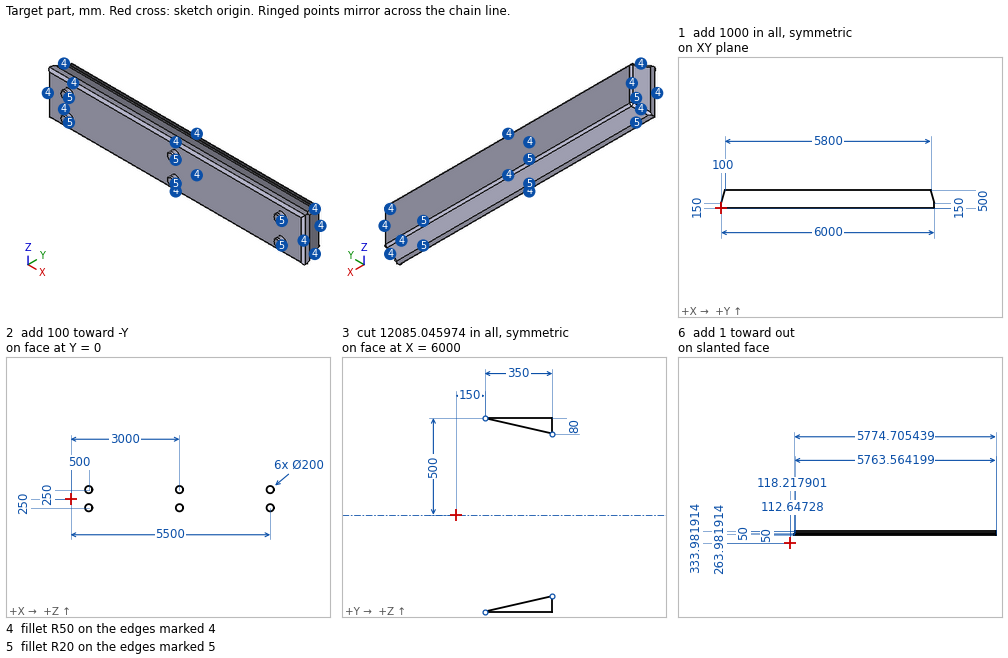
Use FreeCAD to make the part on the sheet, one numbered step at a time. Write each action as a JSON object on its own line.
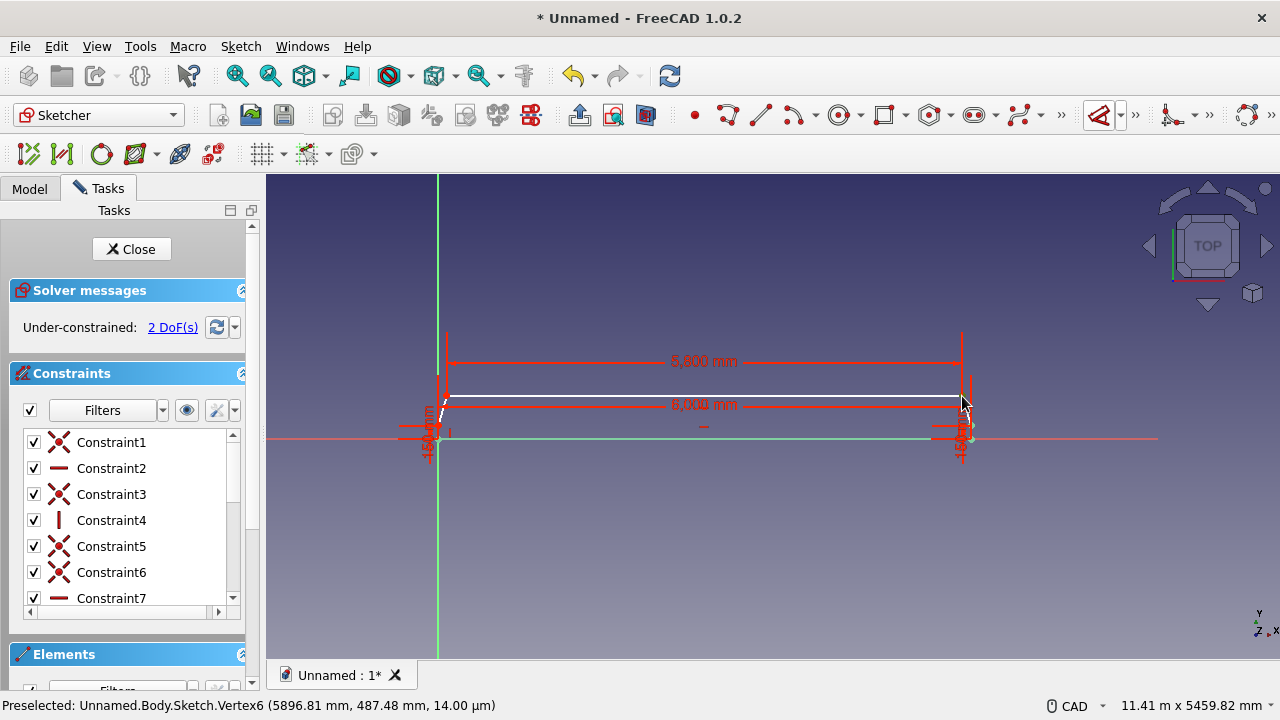
{"action": "left_click", "coordinate": [1120, 116]}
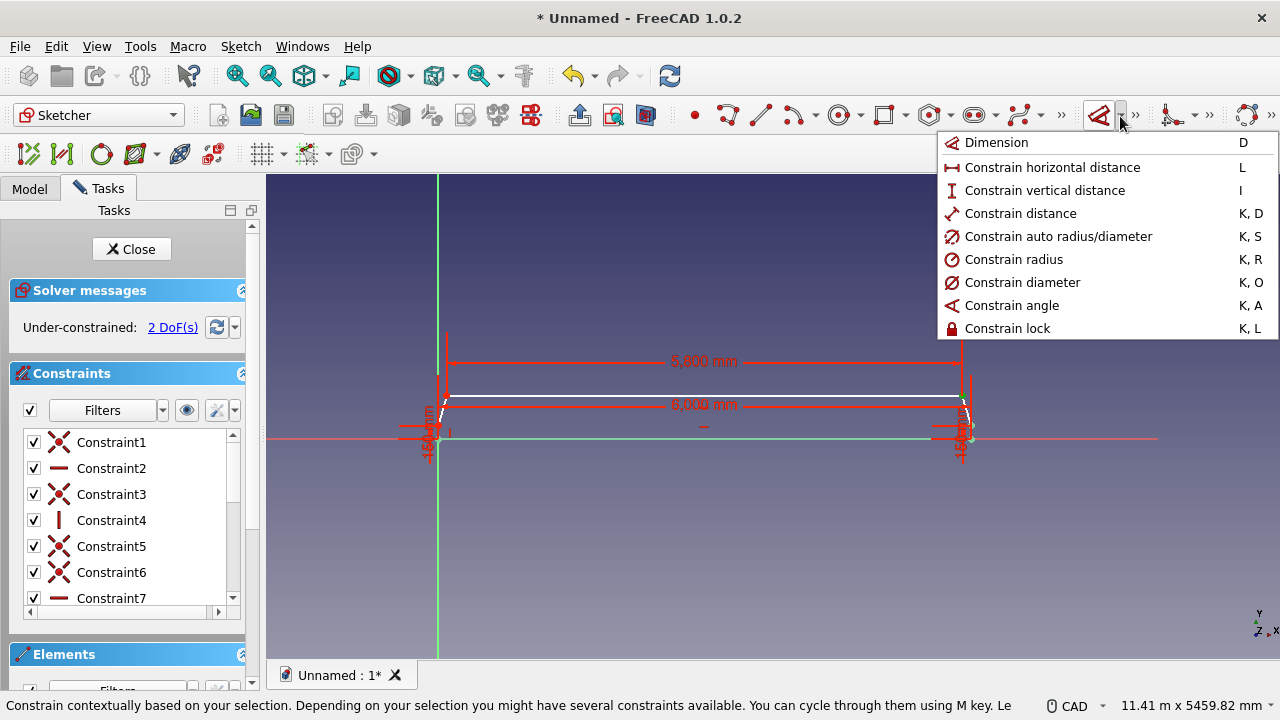
{"action": "left_click", "coordinate": [1108, 190]}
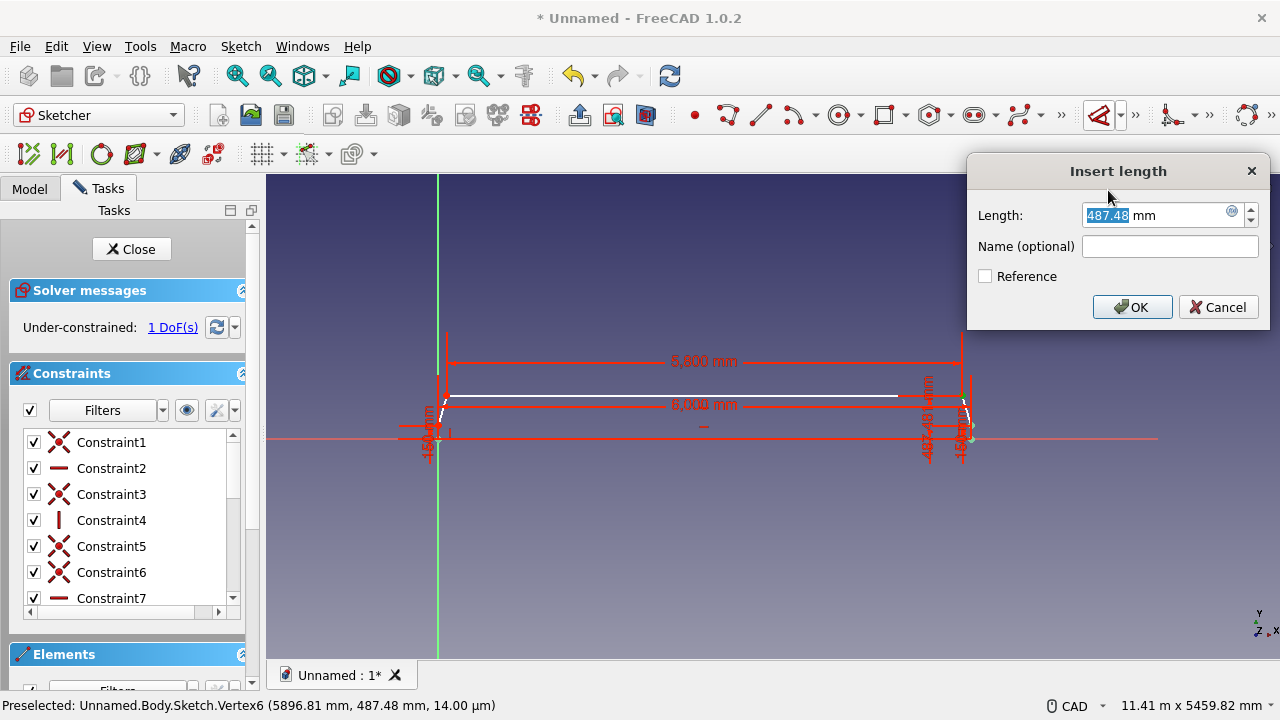
{"action": "type", "text": "500"}
{"action": "key", "text": "Return"}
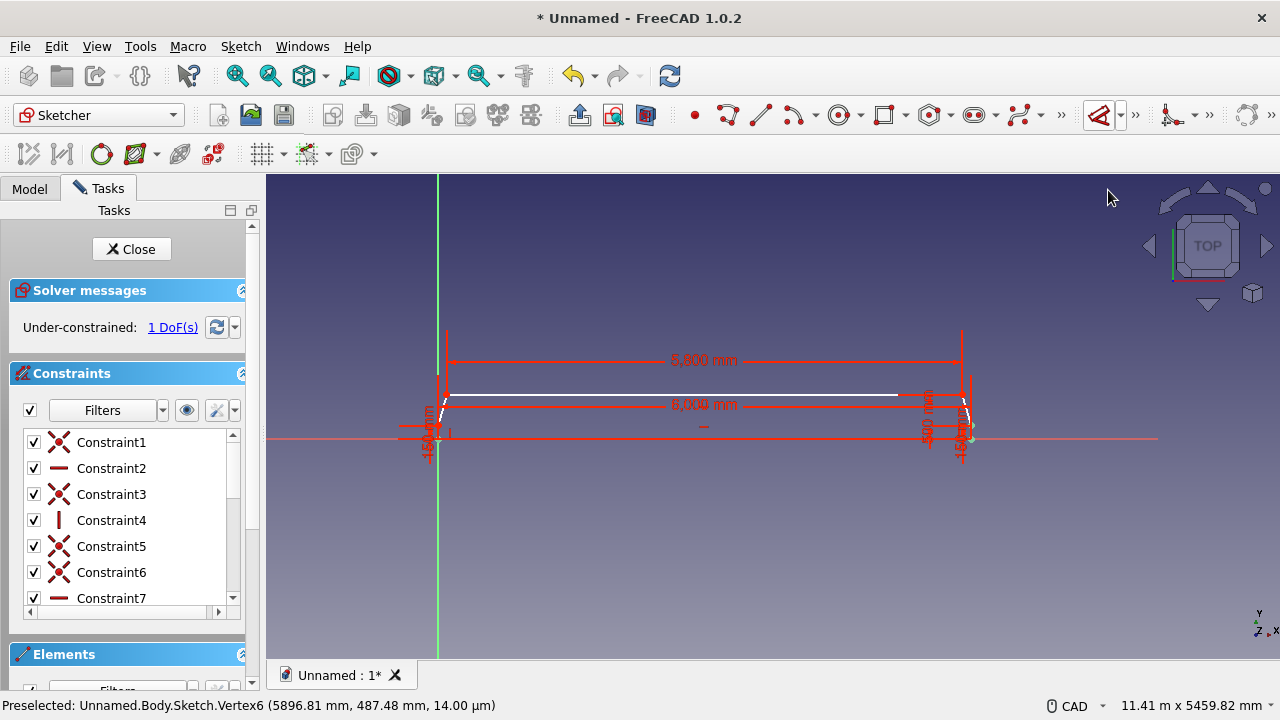
{"action": "scroll", "coordinate": [447, 395], "scroll_direction": "up", "scroll_amount": 8}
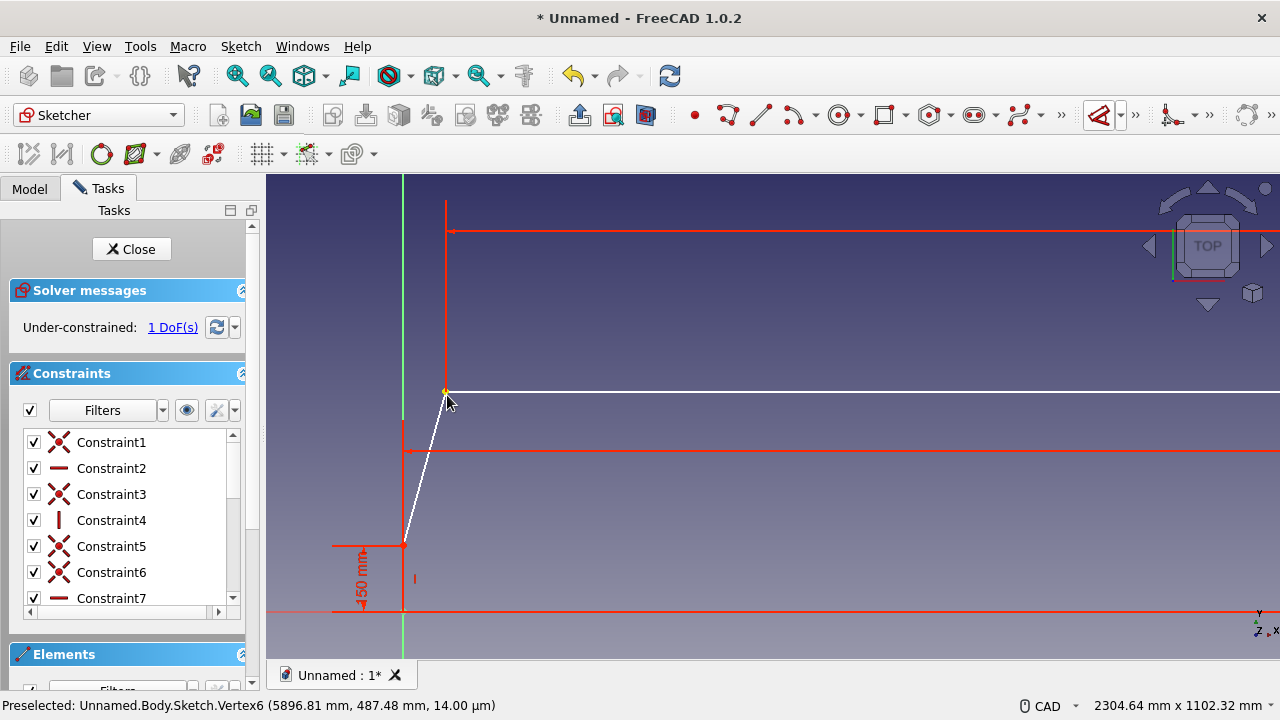
{"action": "left_click", "coordinate": [446, 392]}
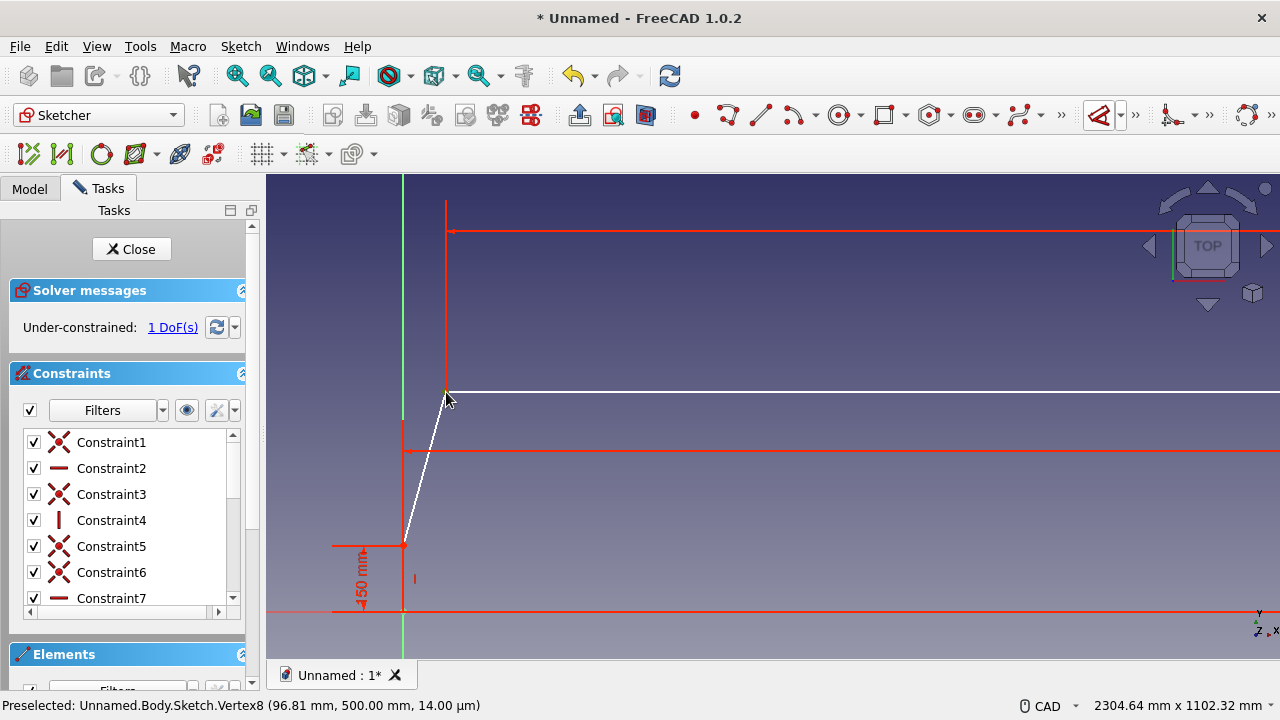
{"action": "key", "text": "l"}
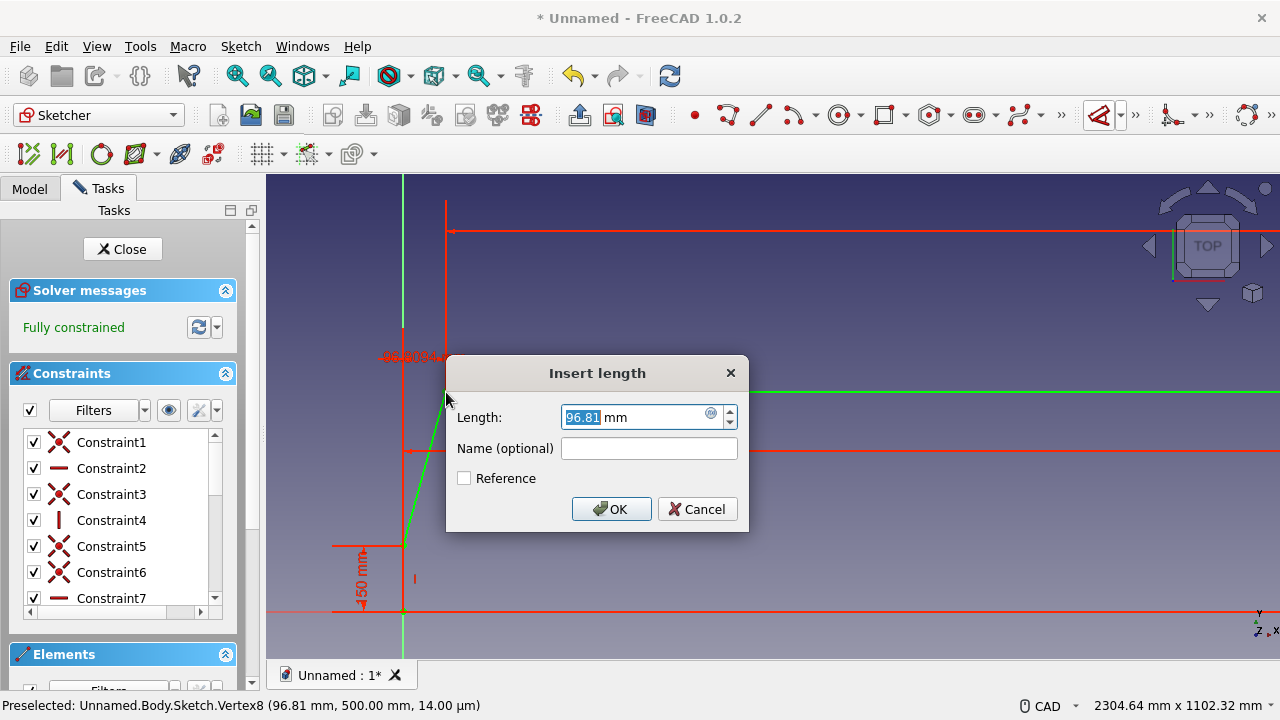
{"action": "type", "text": "100"}
{"action": "key", "text": "Return"}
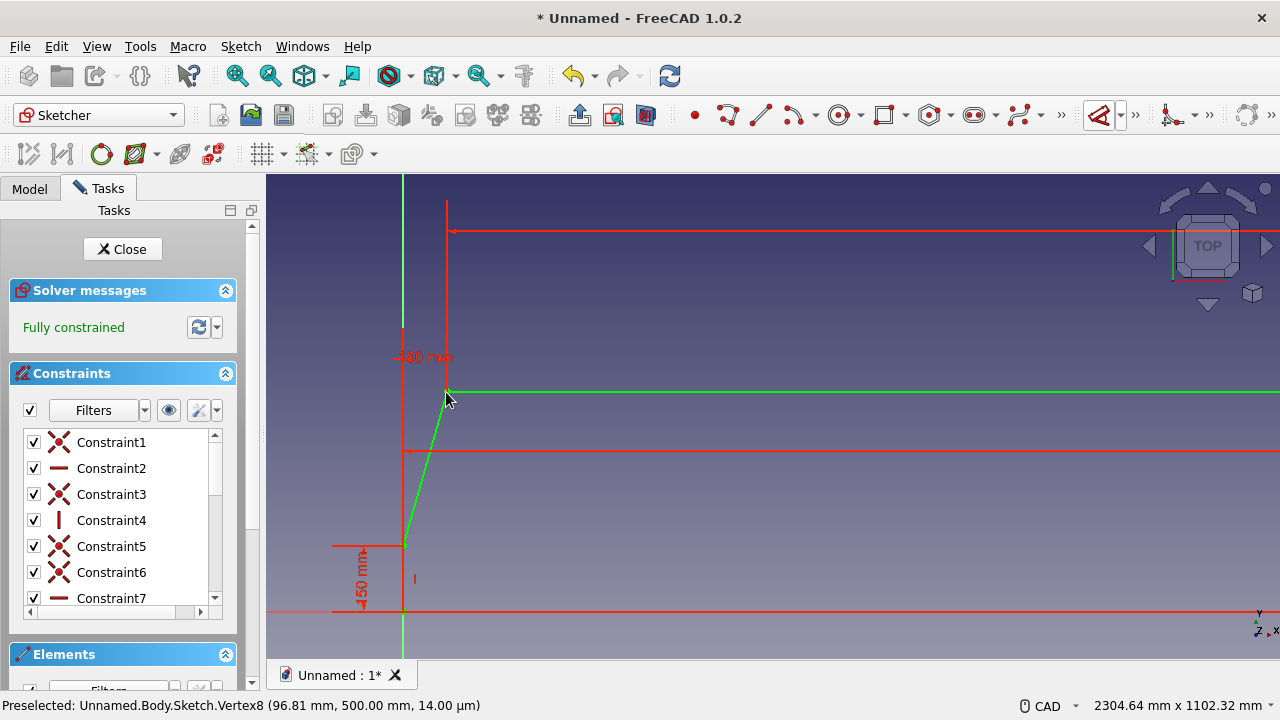
{"action": "left_click", "coordinate": [123, 249]}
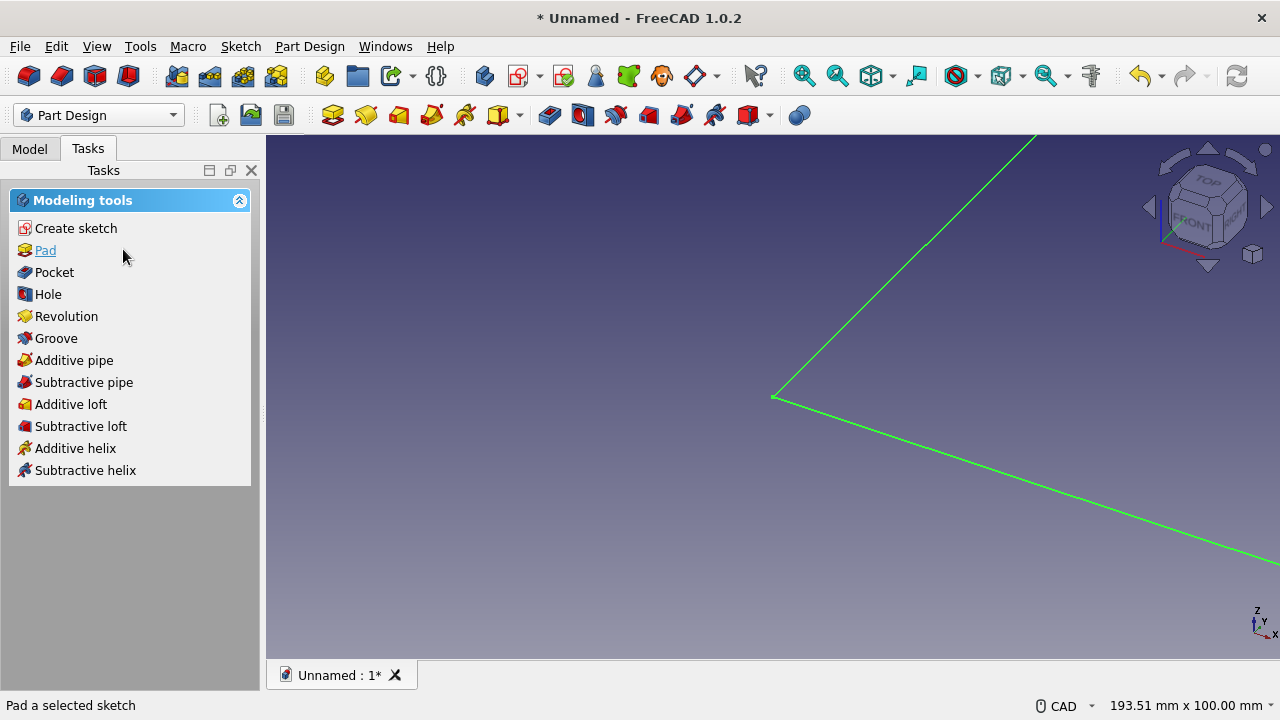
{"action": "left_click", "coordinate": [333, 116]}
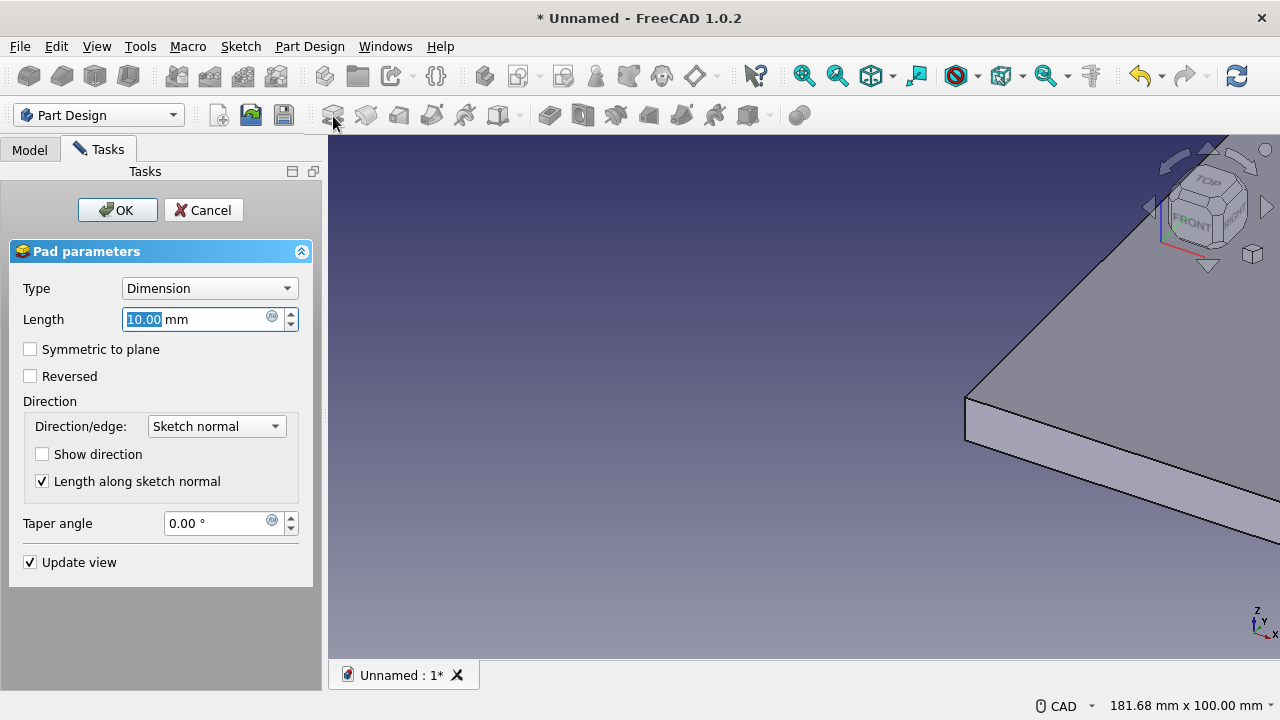
{"action": "type", "text": "1000"}
{"action": "key", "text": "Tab"}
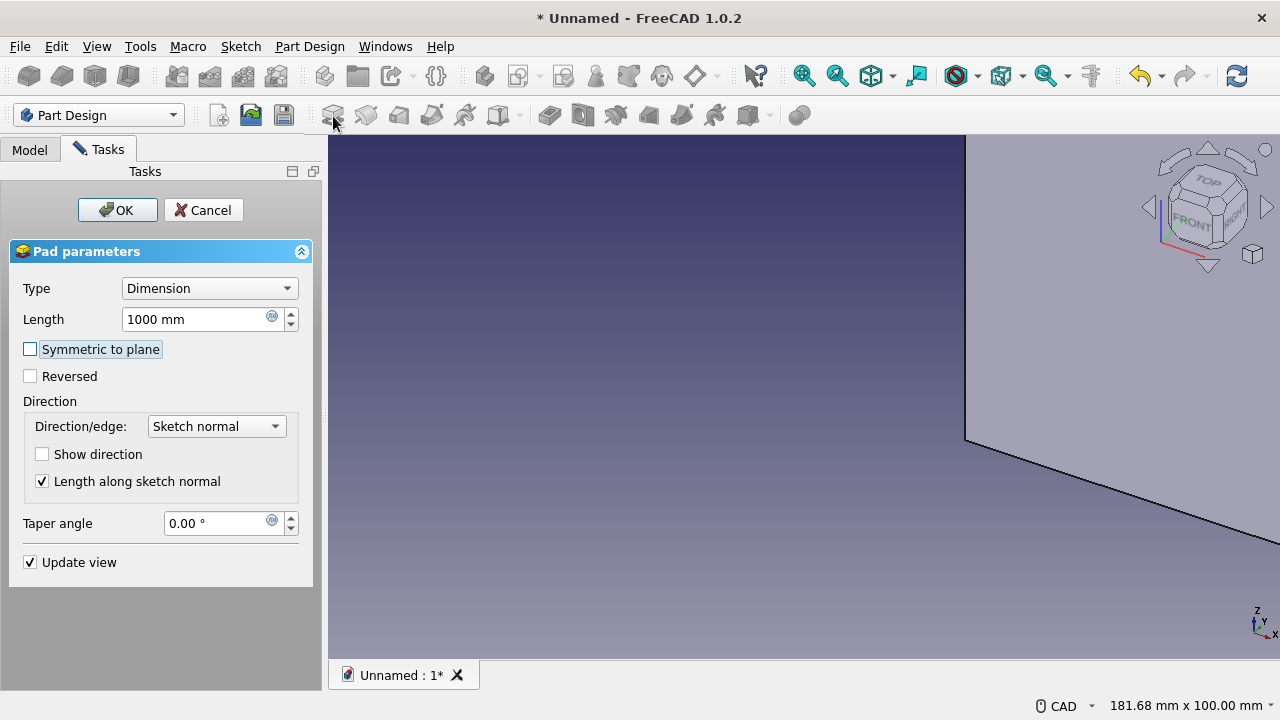
{"action": "left_click", "coordinate": [31, 349]}